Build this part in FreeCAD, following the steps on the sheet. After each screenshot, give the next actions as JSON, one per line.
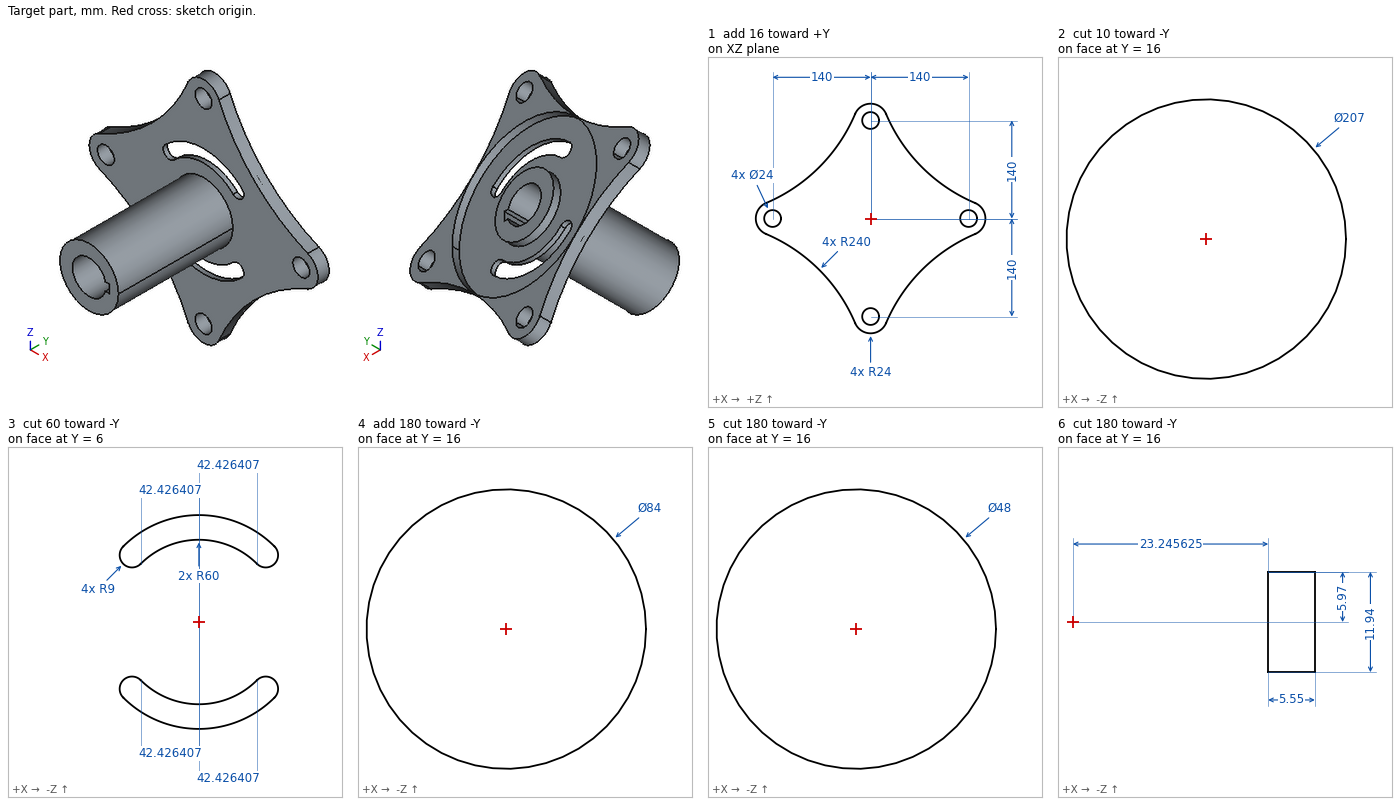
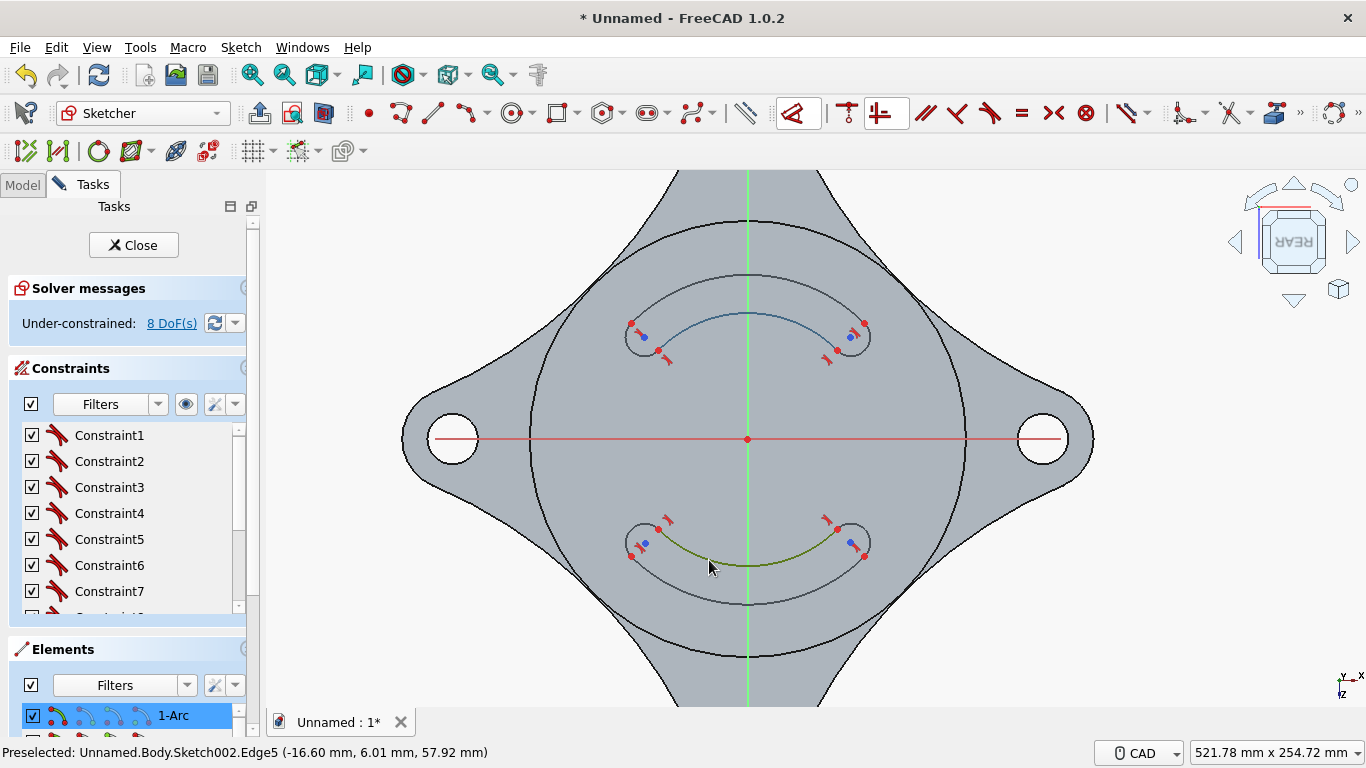
{"action": "left_click", "coordinate": [1022, 114]}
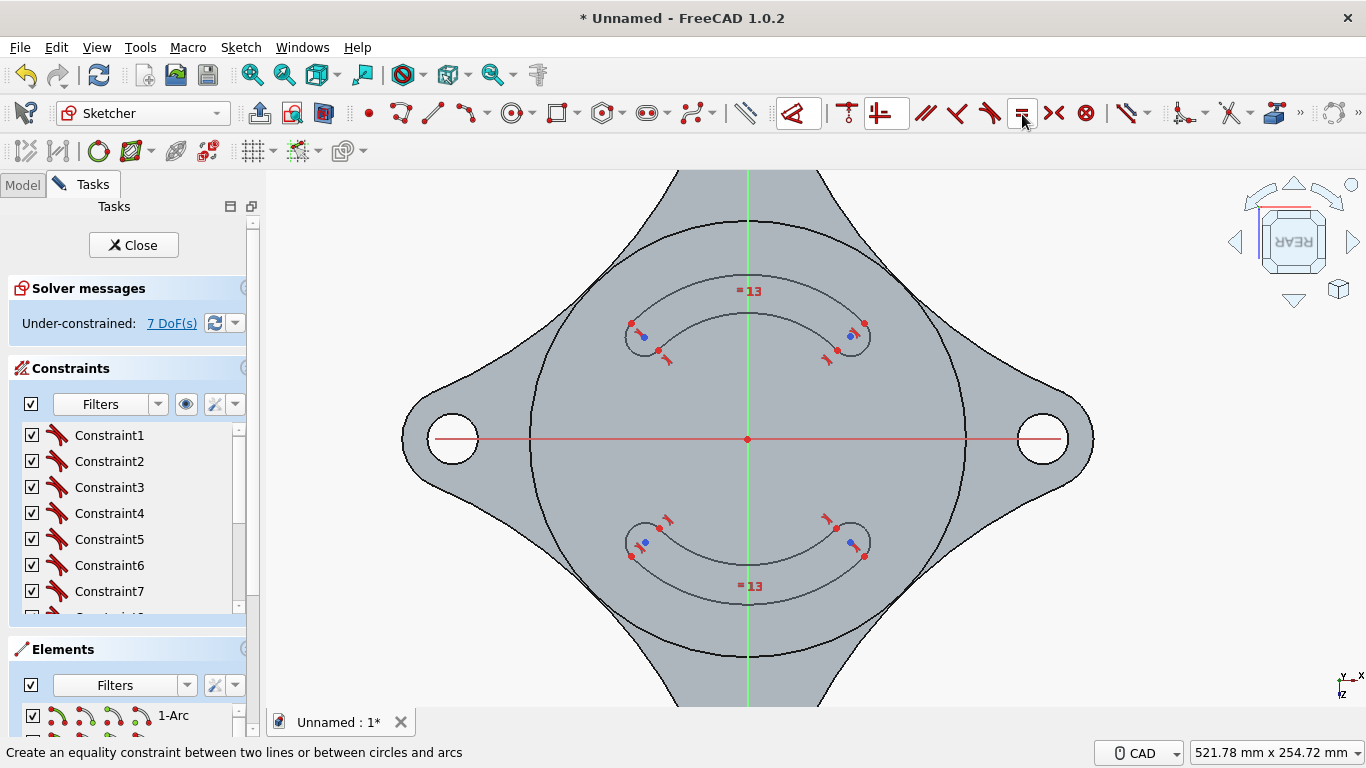
{"action": "left_click", "coordinate": [854, 356]}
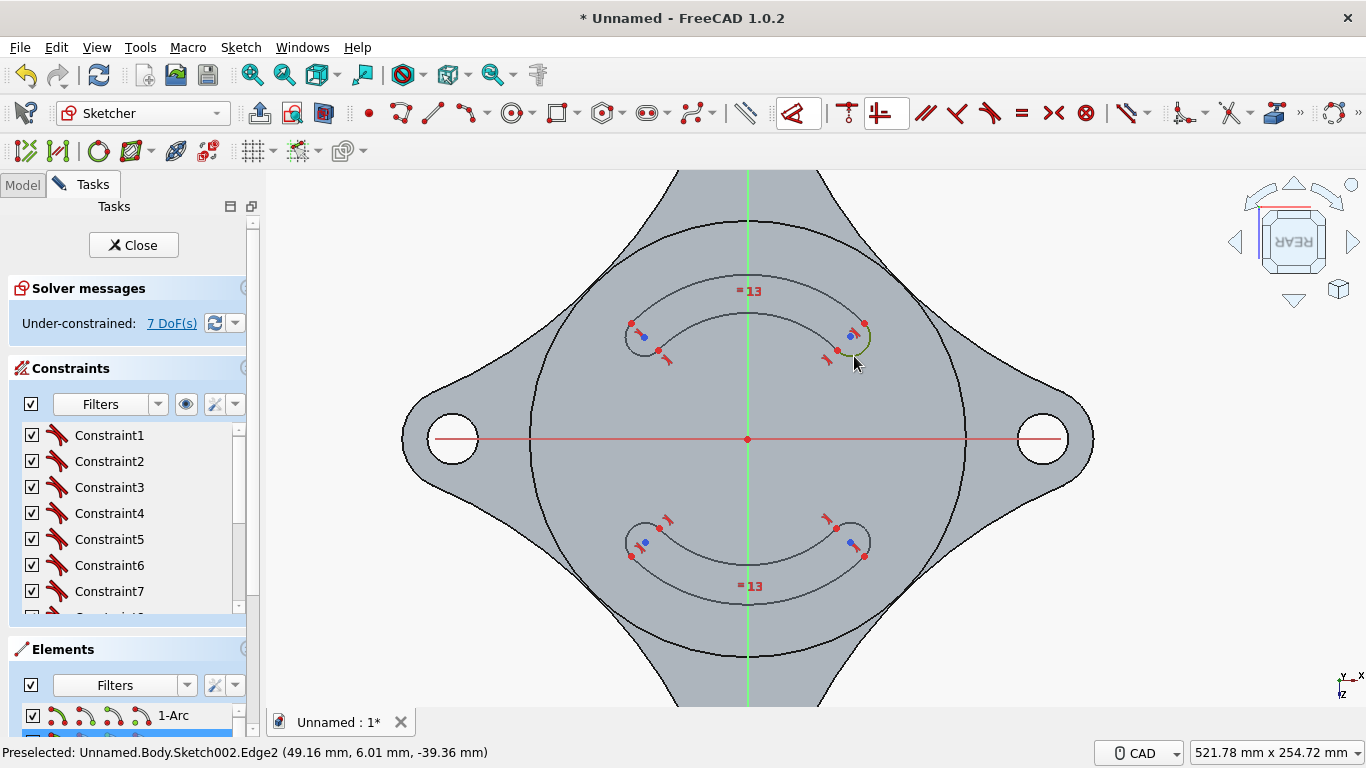
{"action": "left_click", "coordinate": [642, 523]}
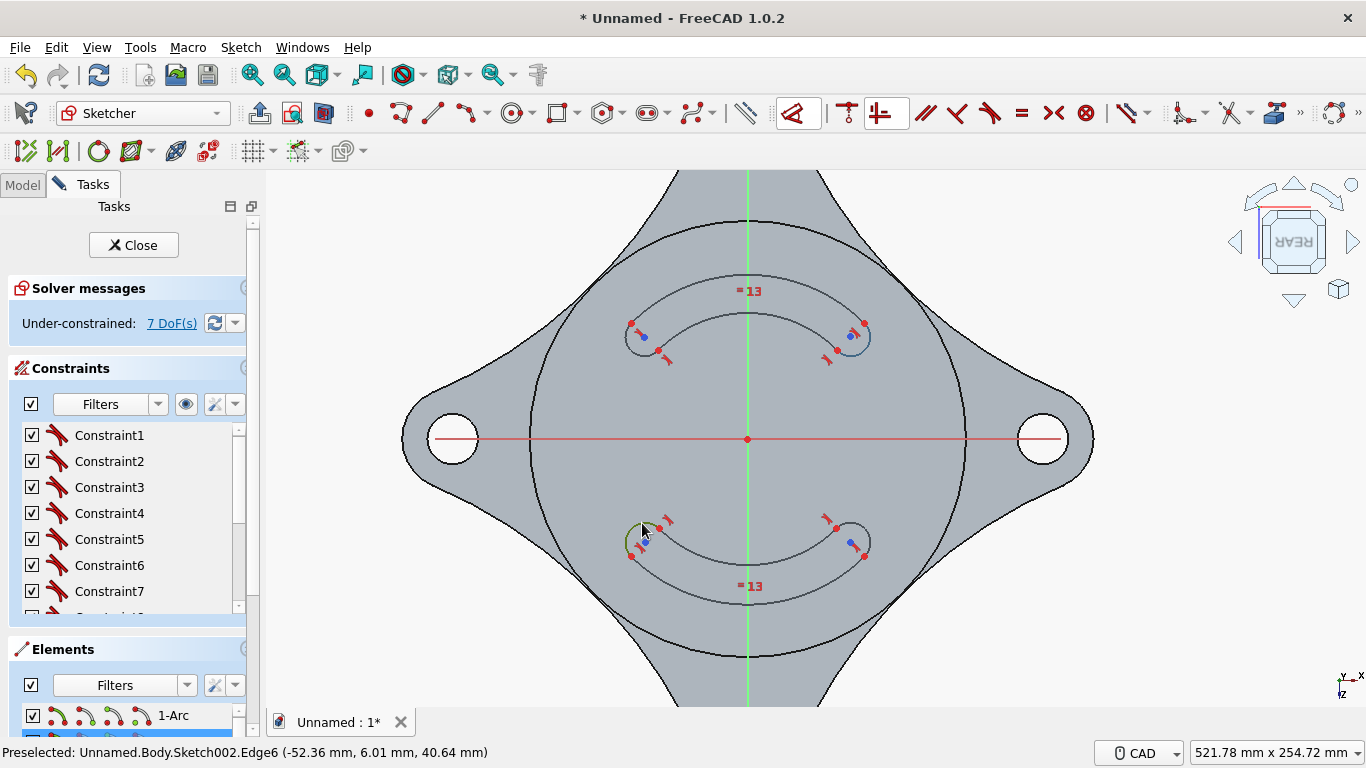
{"action": "left_click", "coordinate": [1022, 114]}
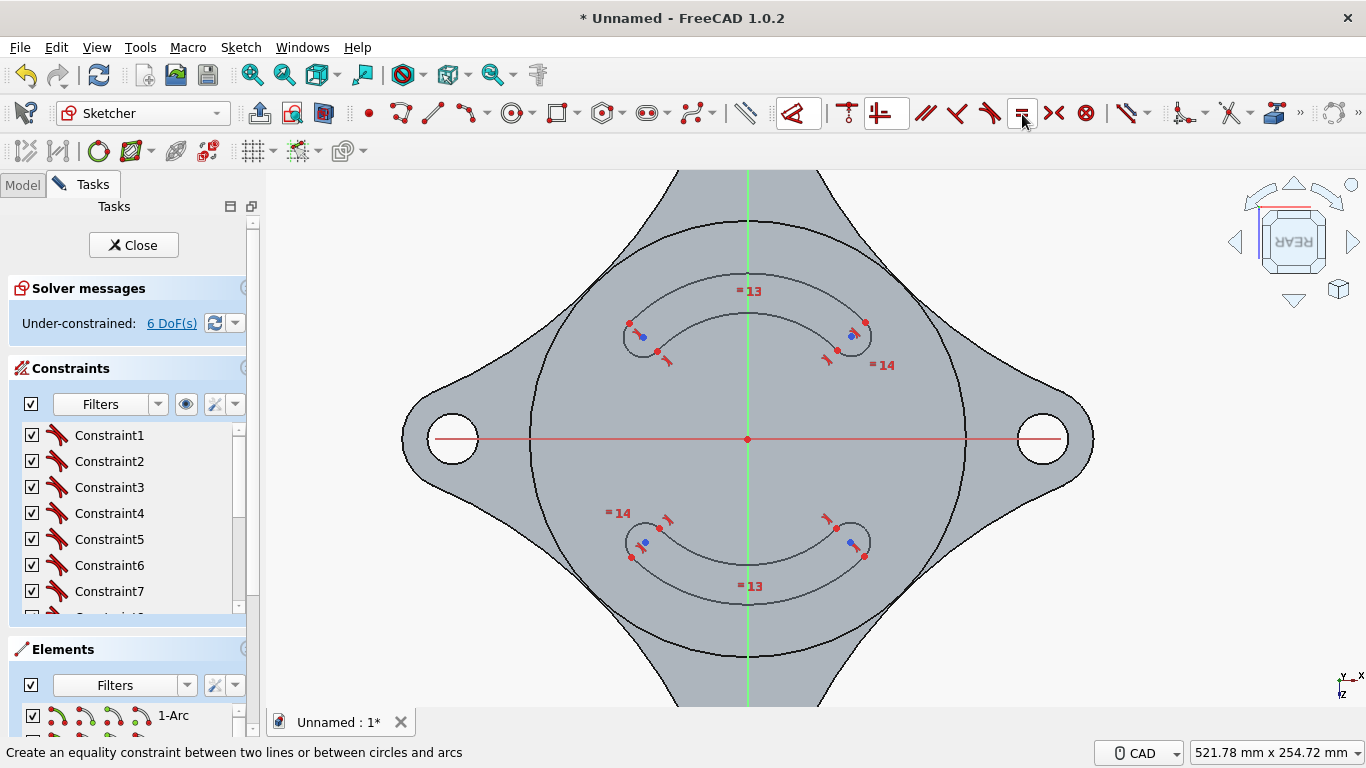
{"action": "left_click", "coordinate": [787, 319]}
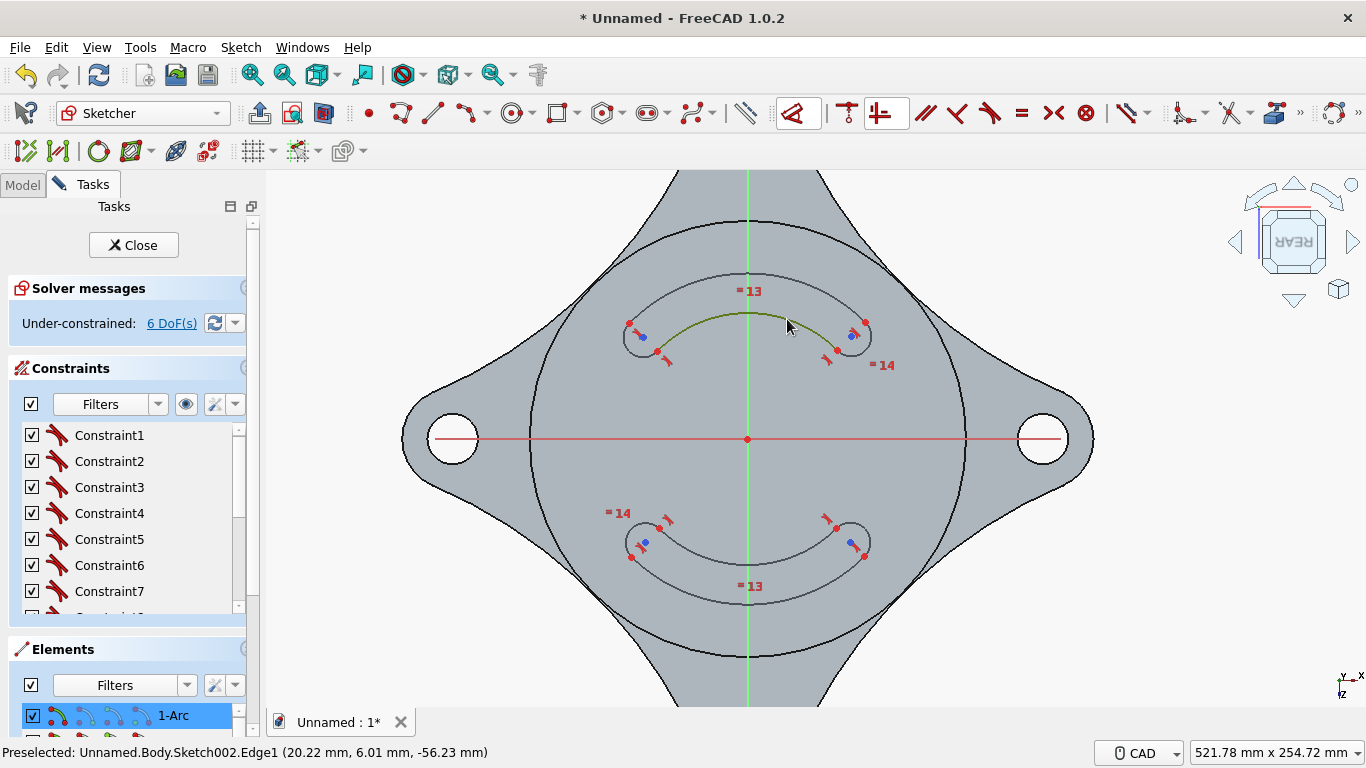
{"action": "key", "text": "k r"}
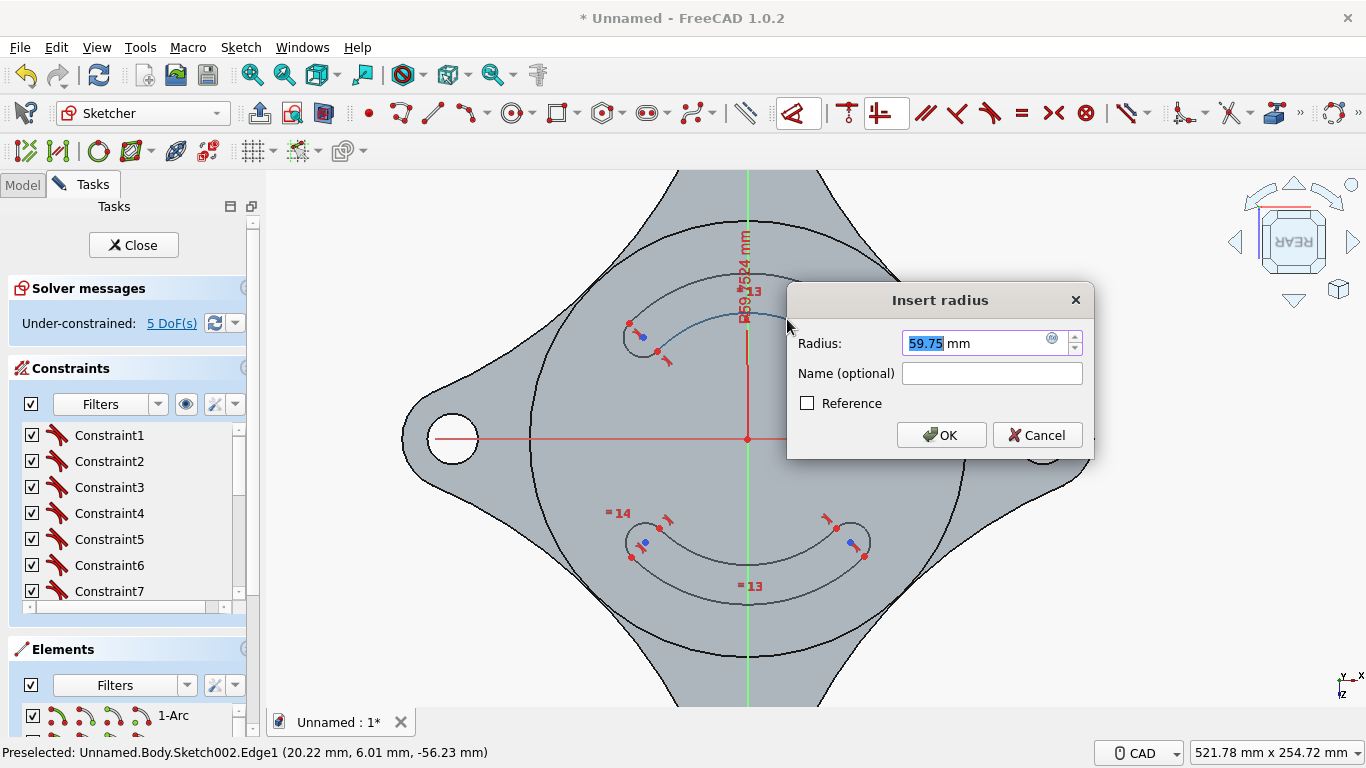
{"action": "type", "text": "60"}
{"action": "key", "text": "Return"}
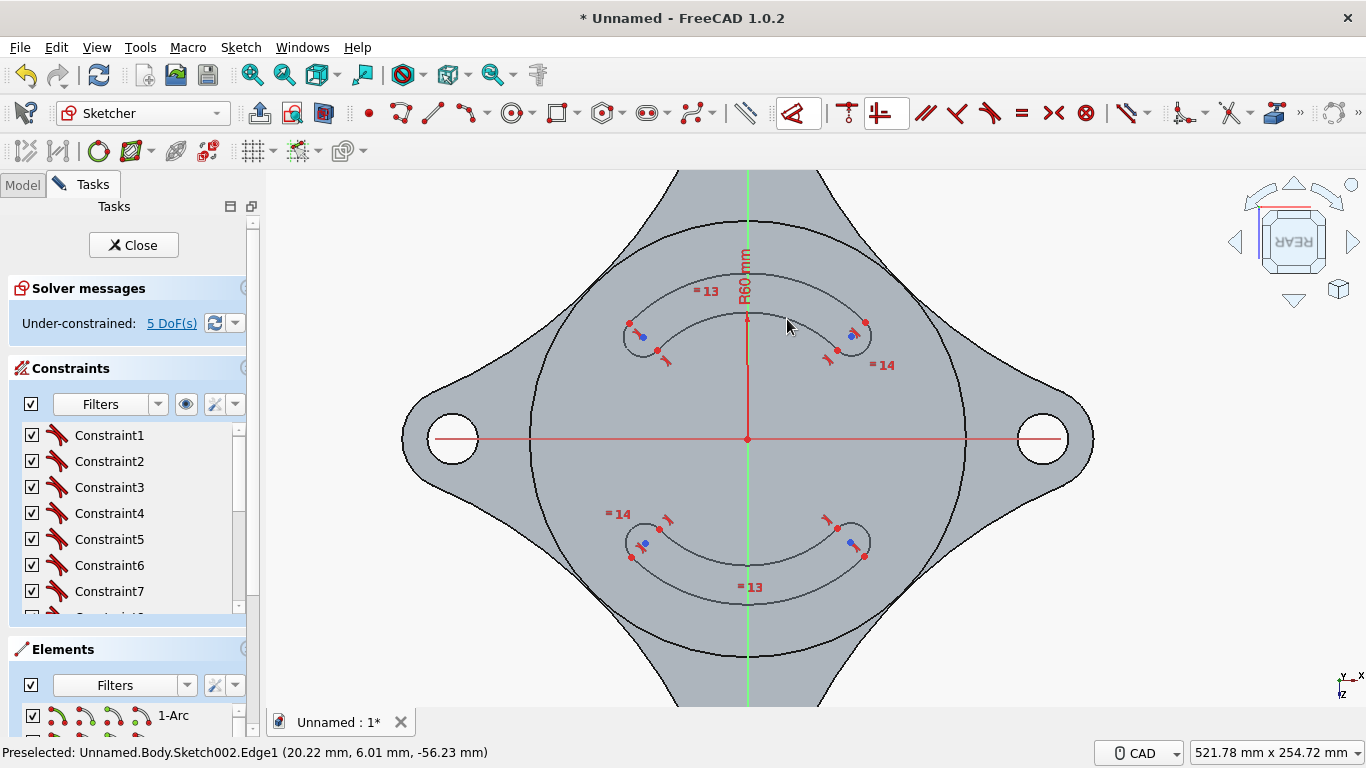
{"action": "scroll", "coordinate": [855, 356], "scroll_direction": "up", "scroll_amount": 4}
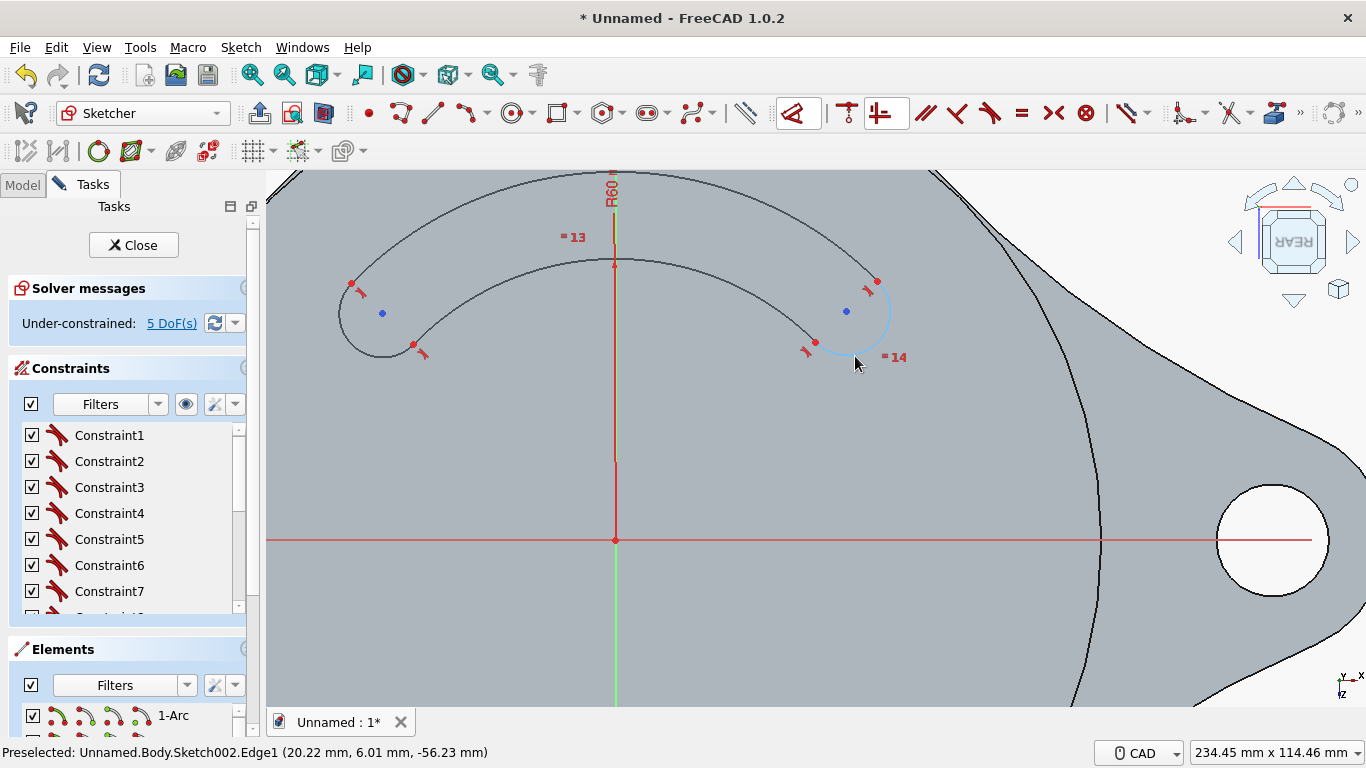
{"action": "left_click", "coordinate": [853, 355]}